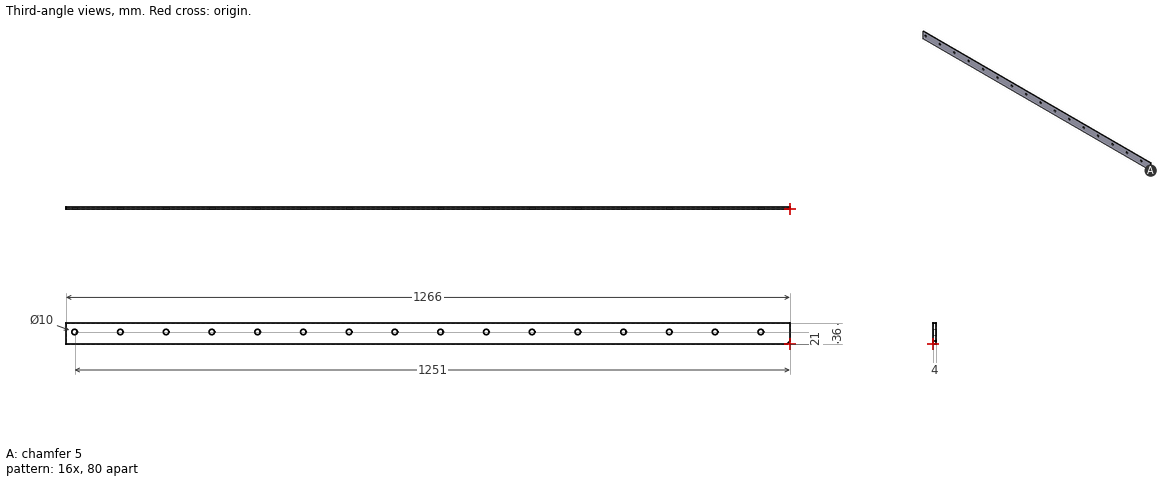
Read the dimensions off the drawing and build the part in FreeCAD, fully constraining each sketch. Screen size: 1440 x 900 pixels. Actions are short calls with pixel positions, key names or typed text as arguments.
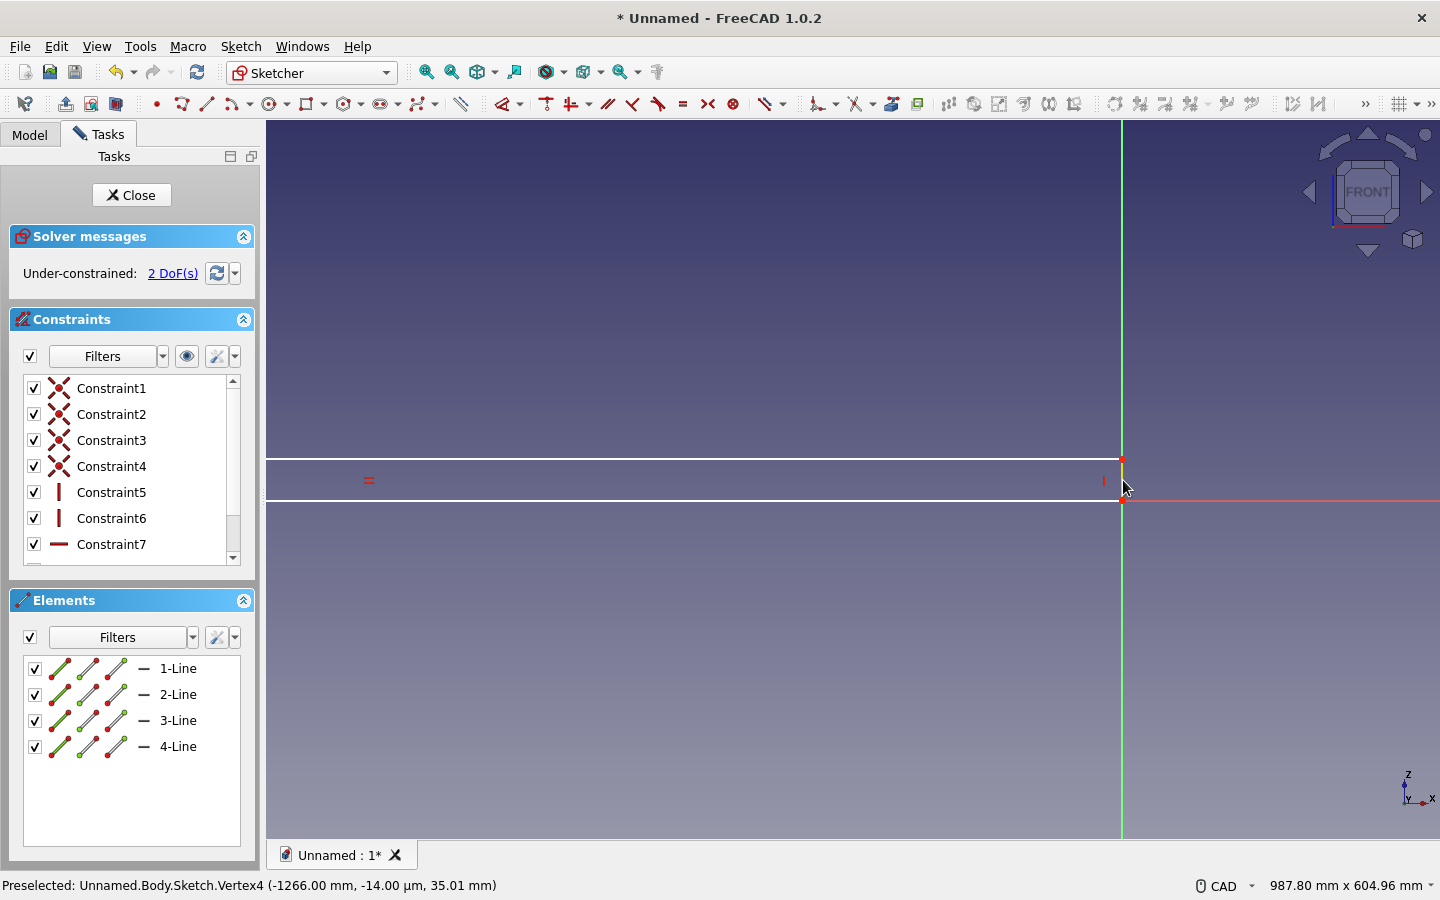
click(1122, 480)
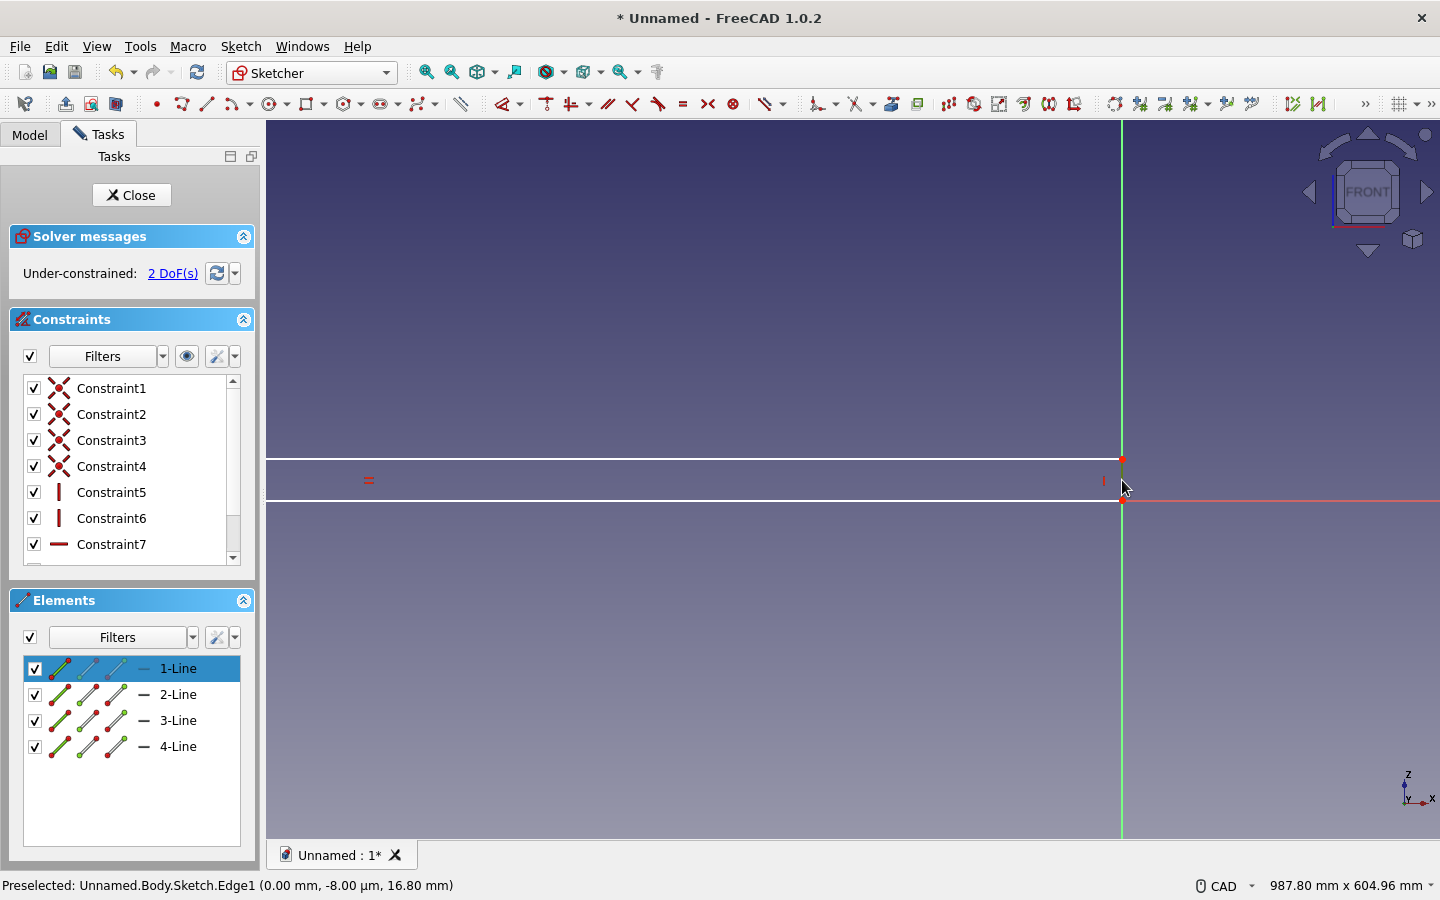
click(520, 104)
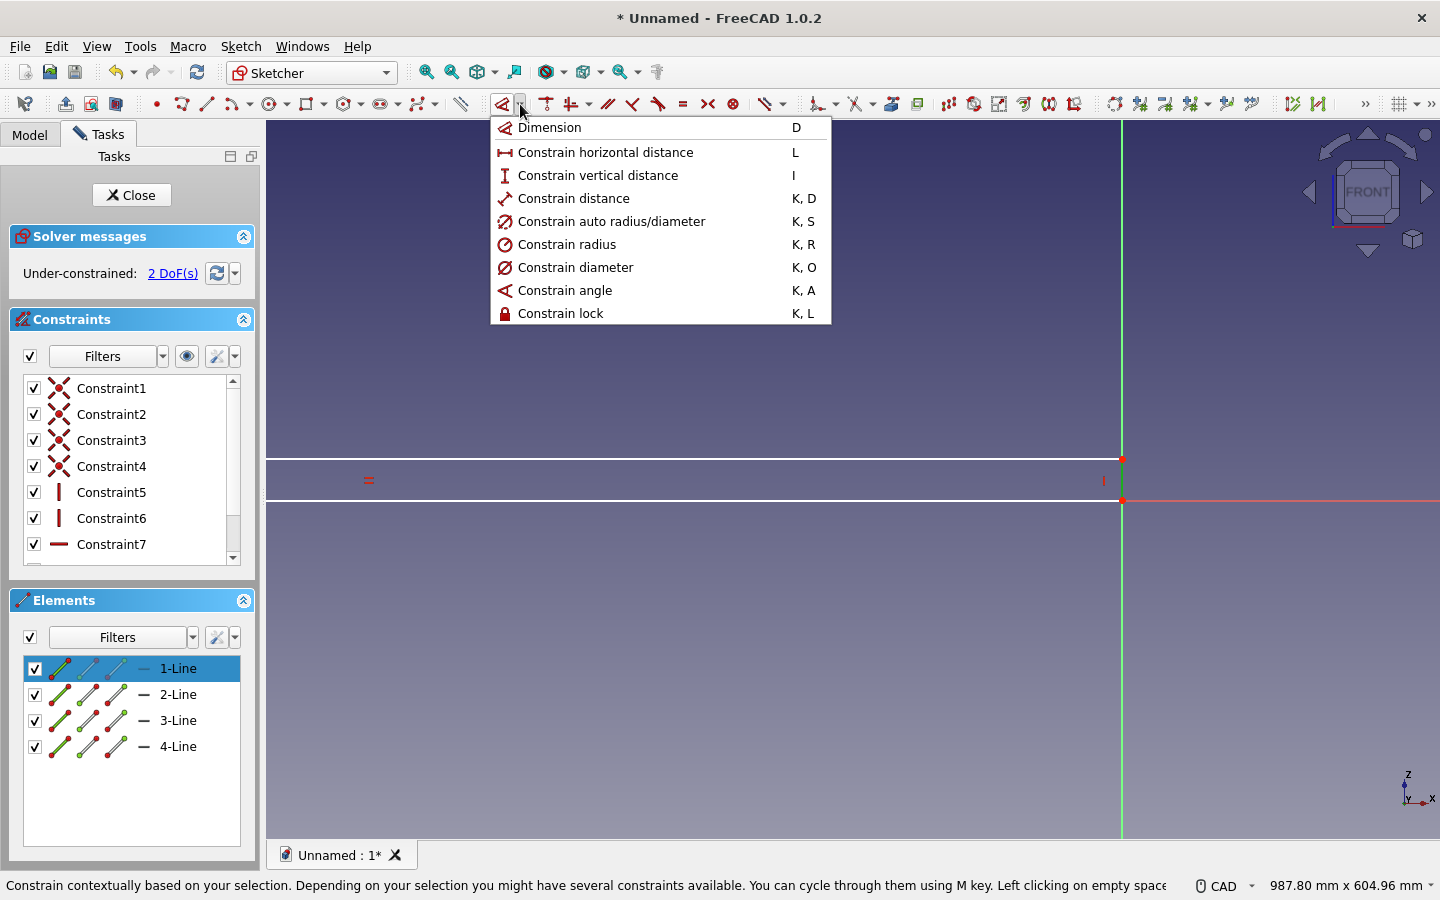
click(661, 176)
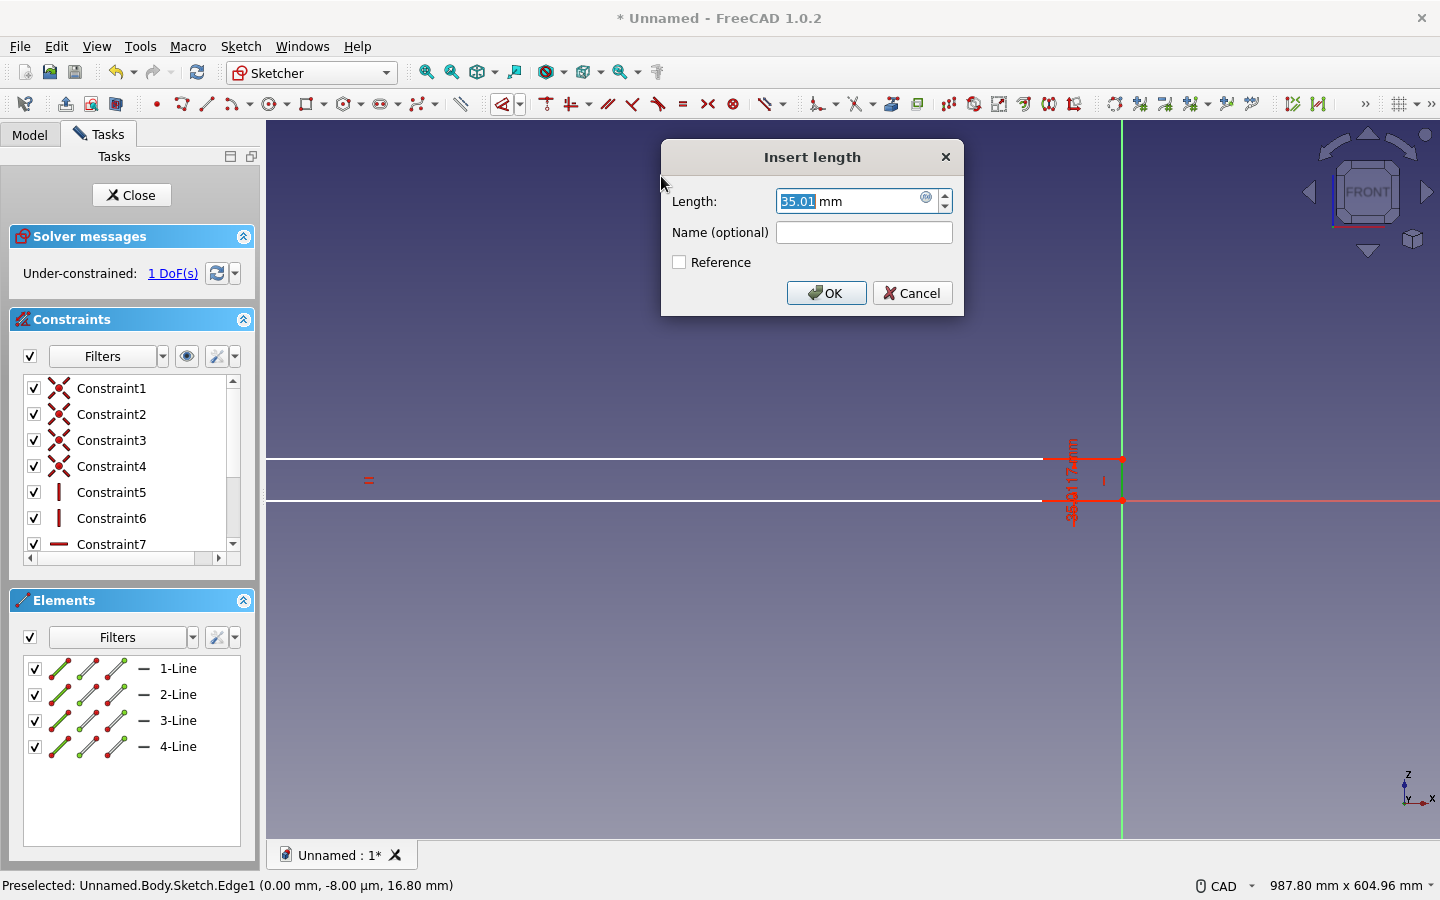
text(36)
key(Return)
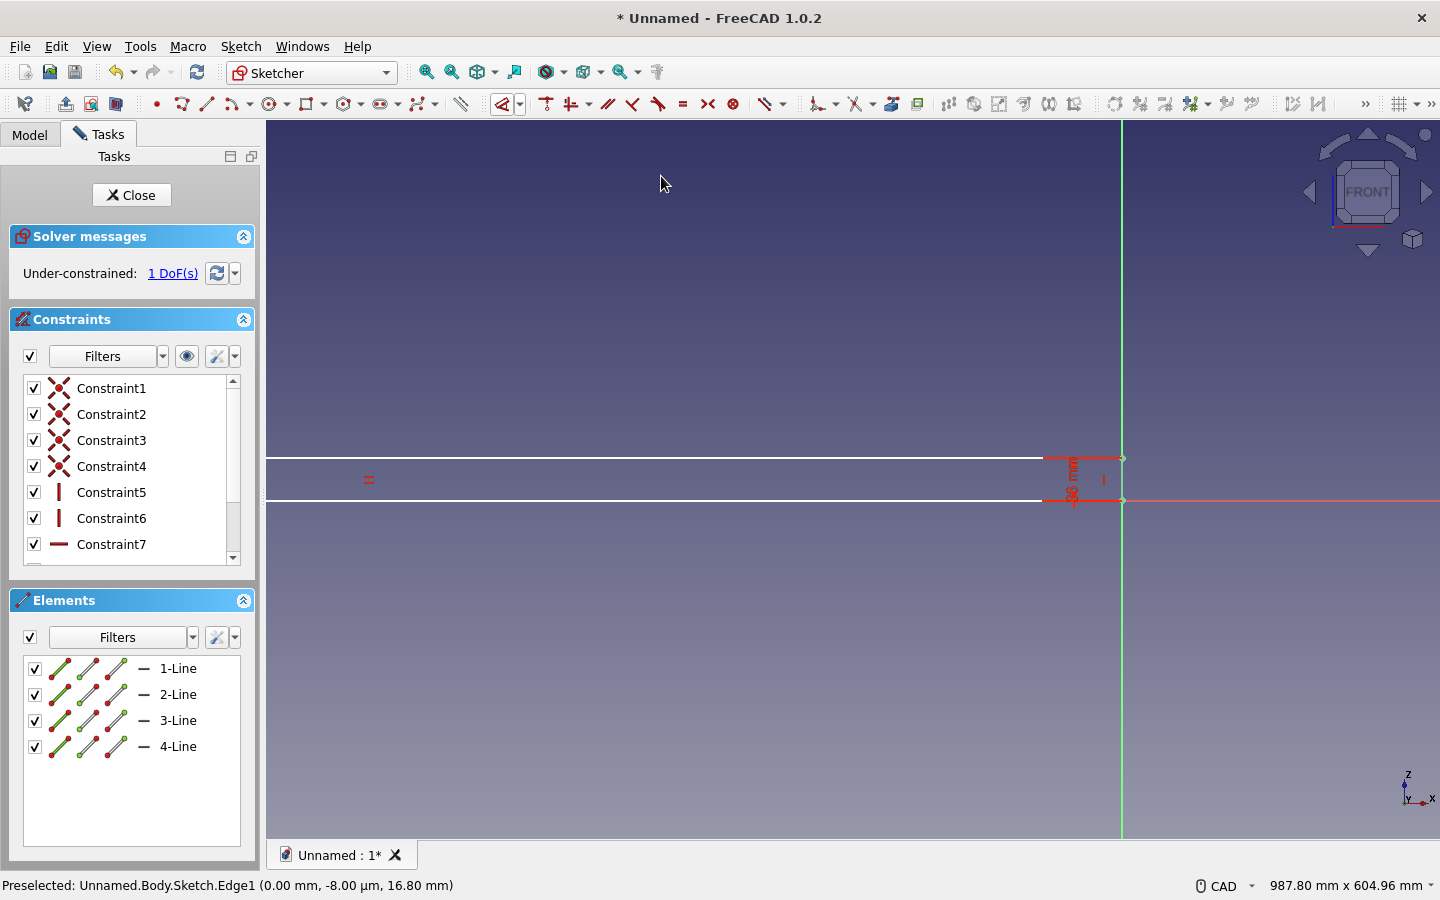
click(671, 458)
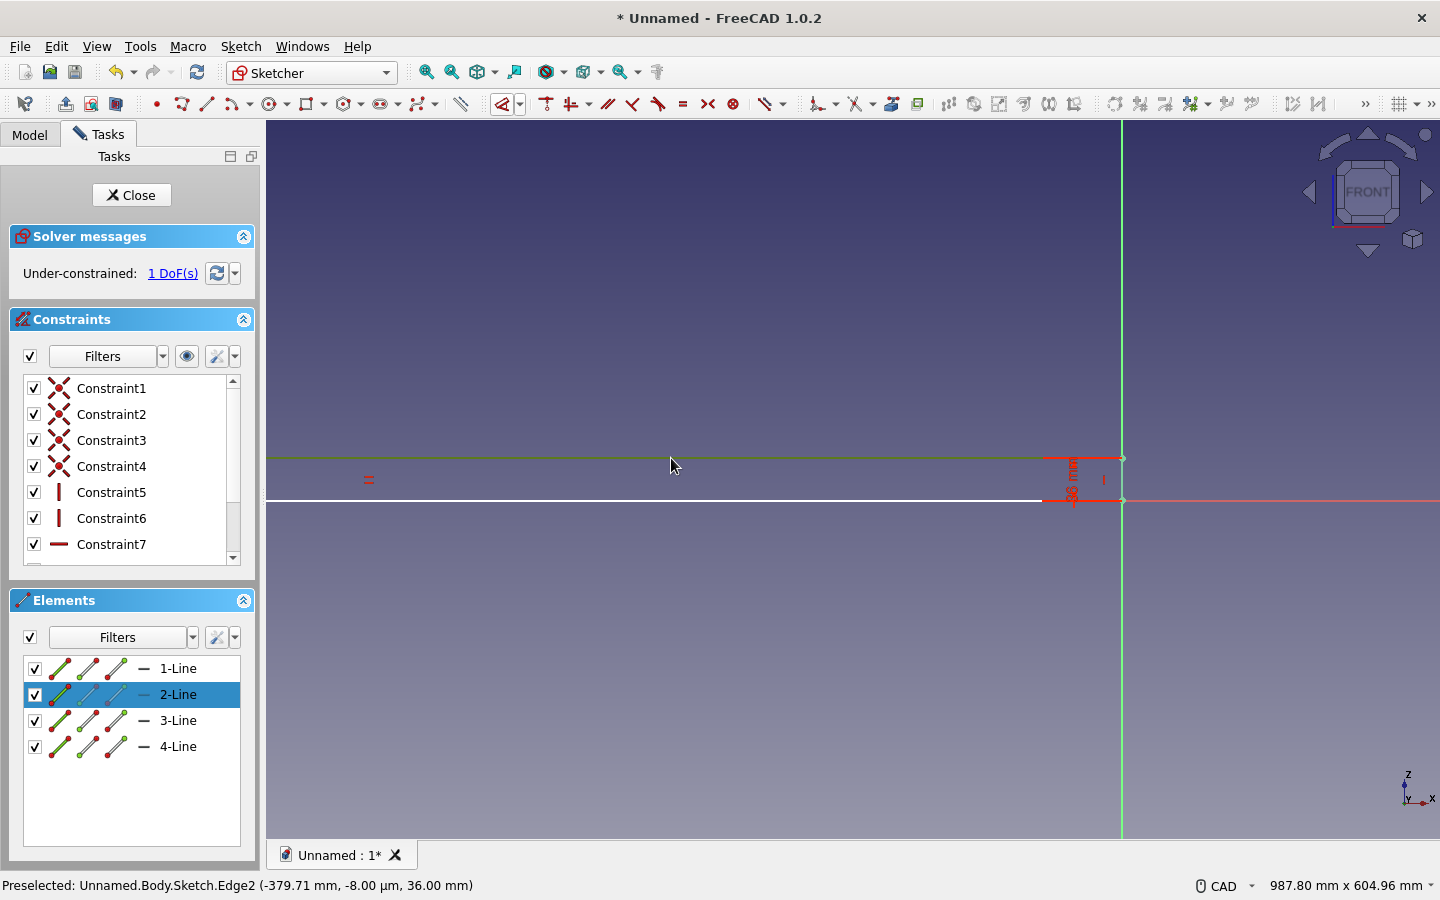
key(l)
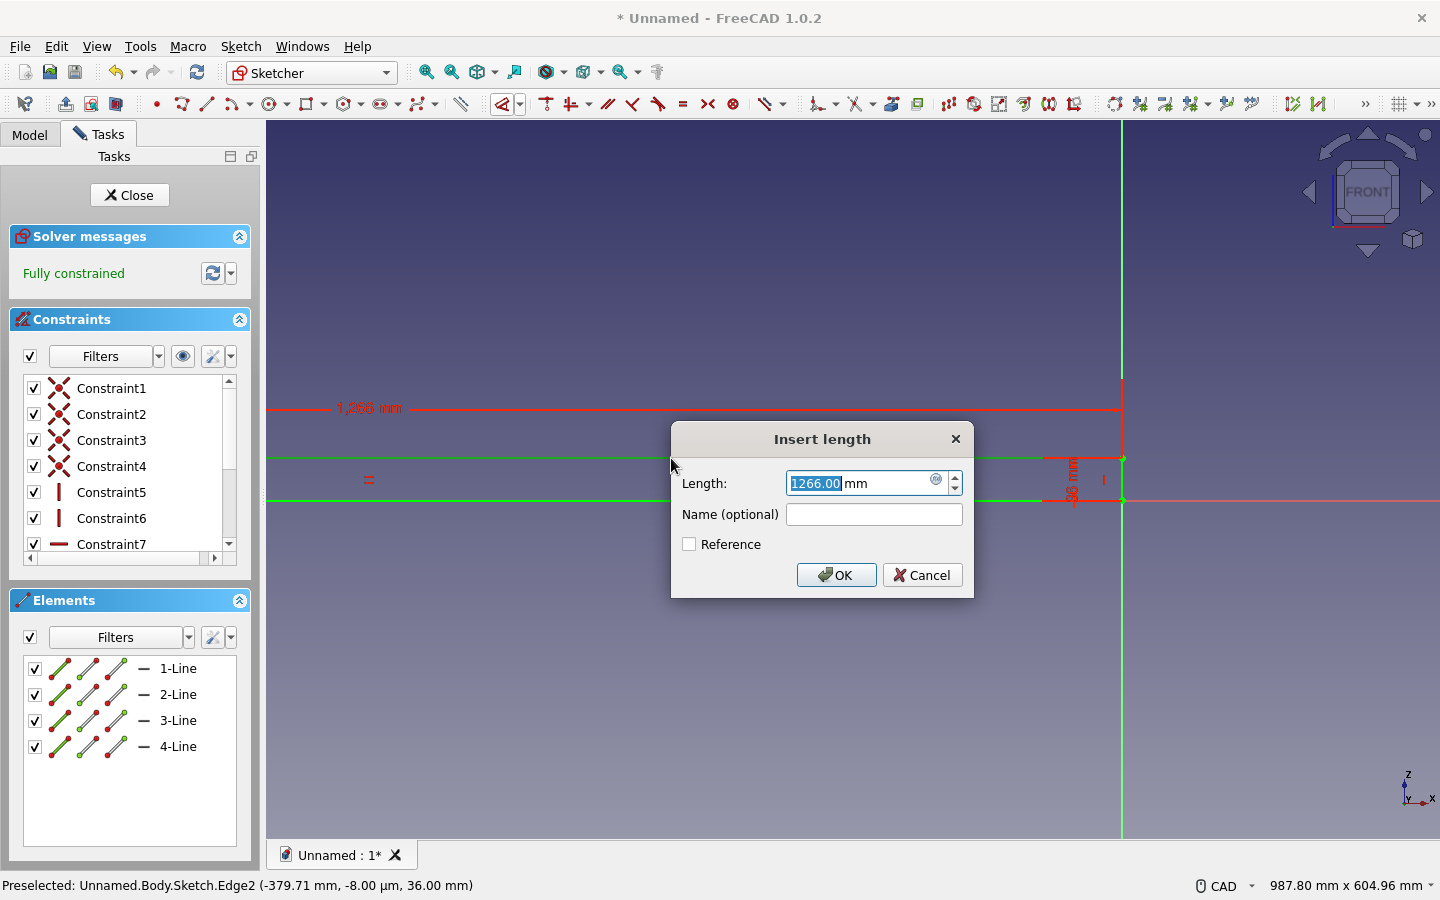
text(1266)
key(Return)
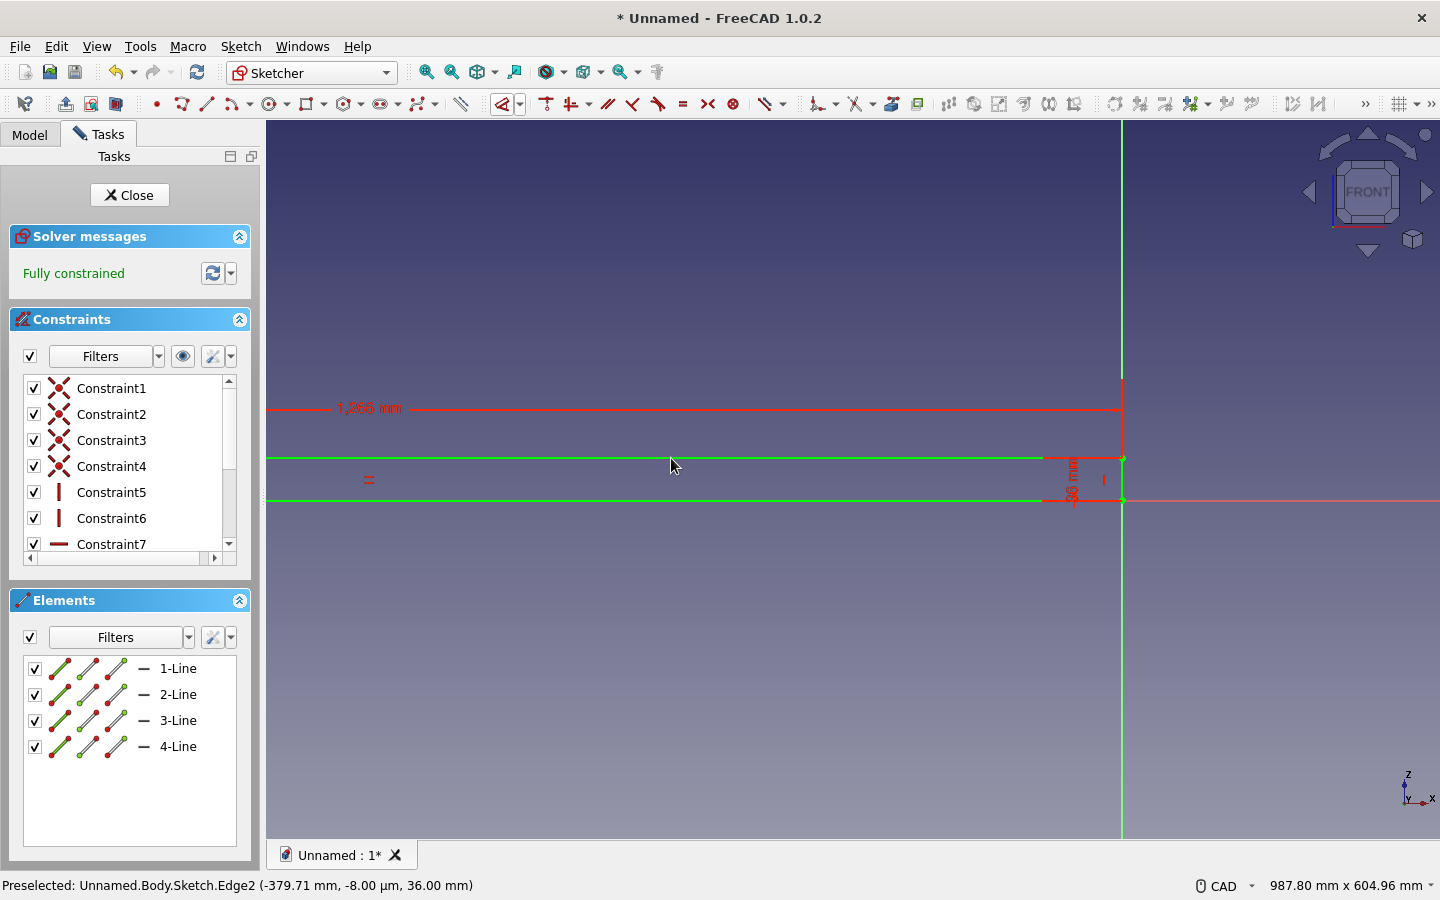
click(130, 195)